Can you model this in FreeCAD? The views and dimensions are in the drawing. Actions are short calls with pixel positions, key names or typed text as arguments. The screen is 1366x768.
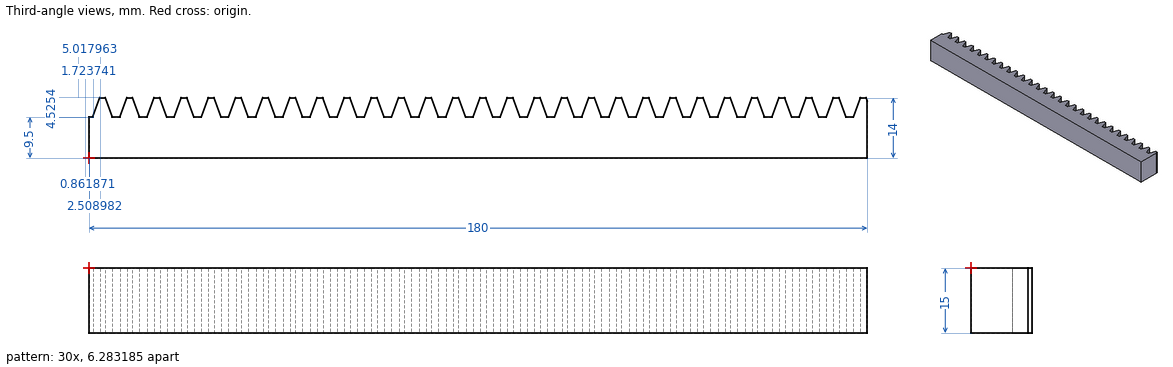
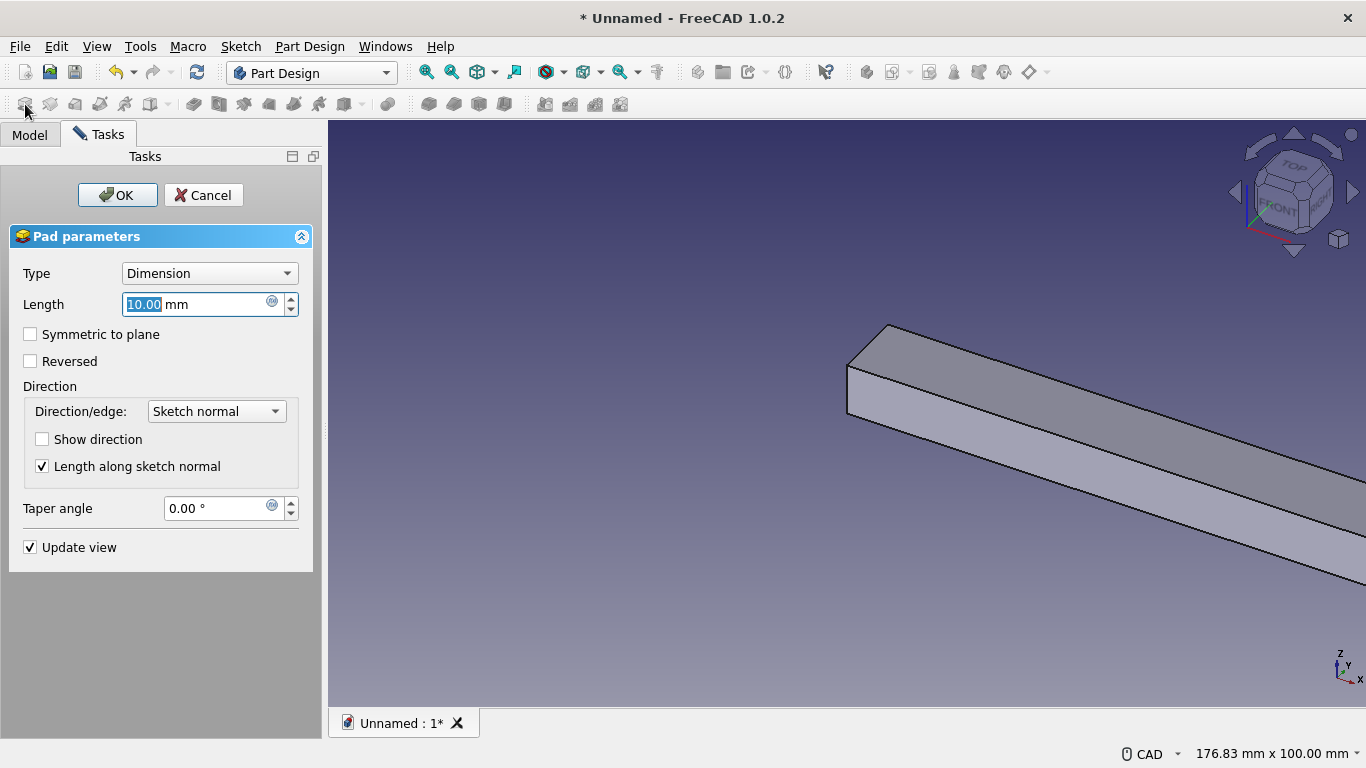
text(15)
key(Tab)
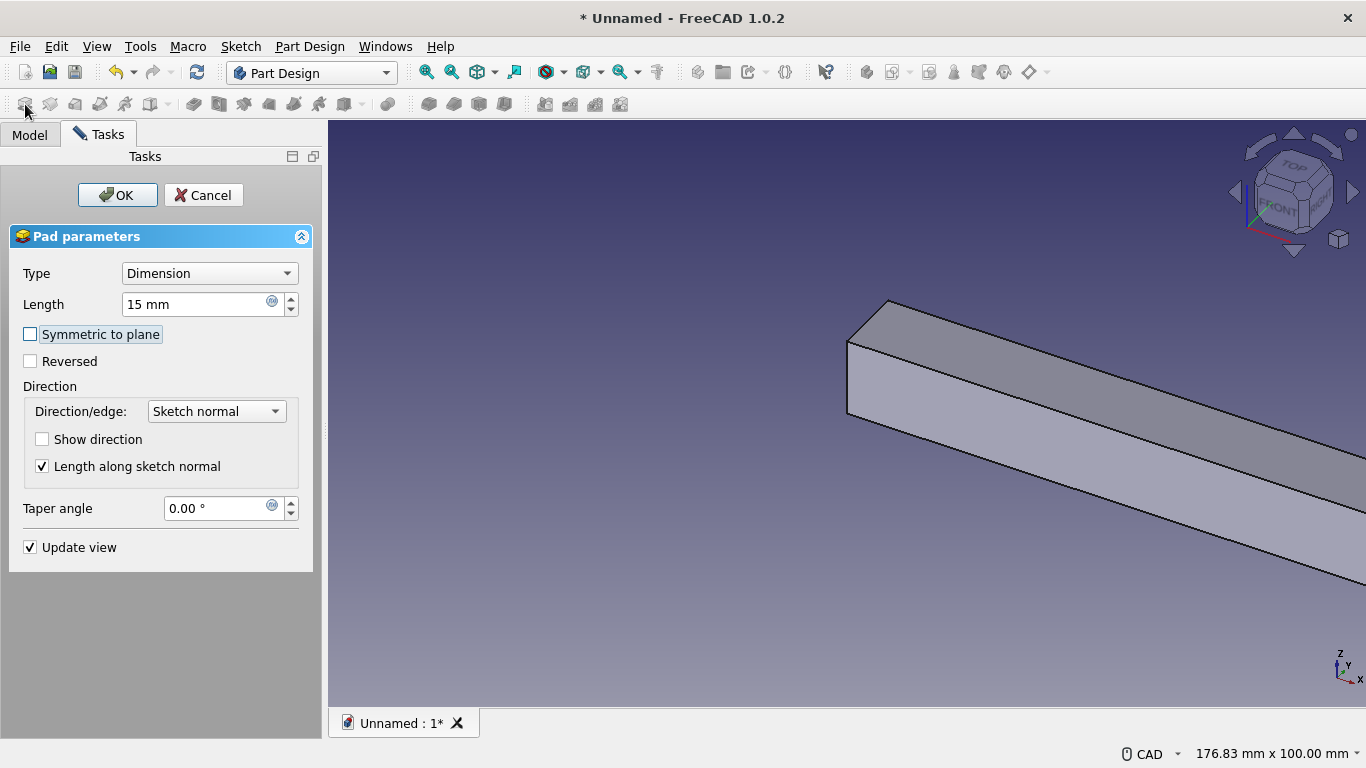
click(31, 361)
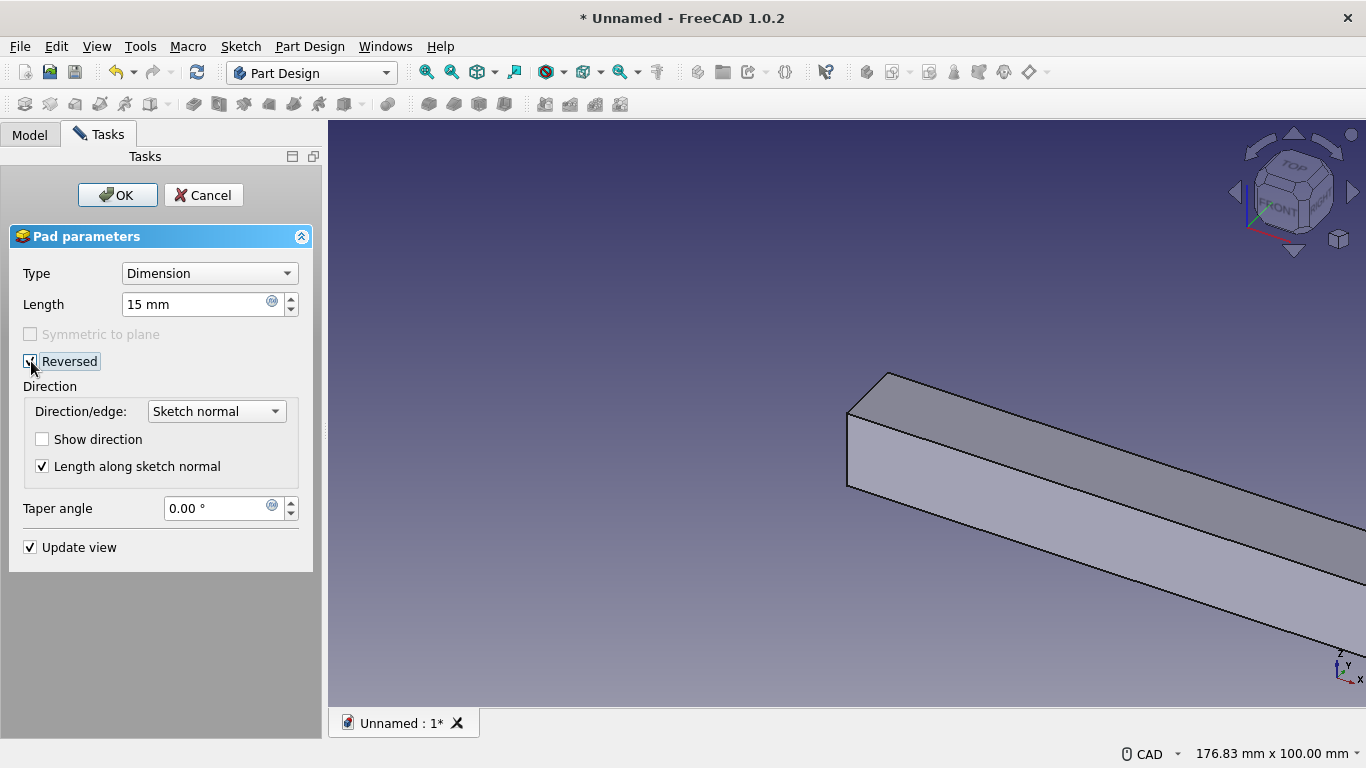
click(118, 195)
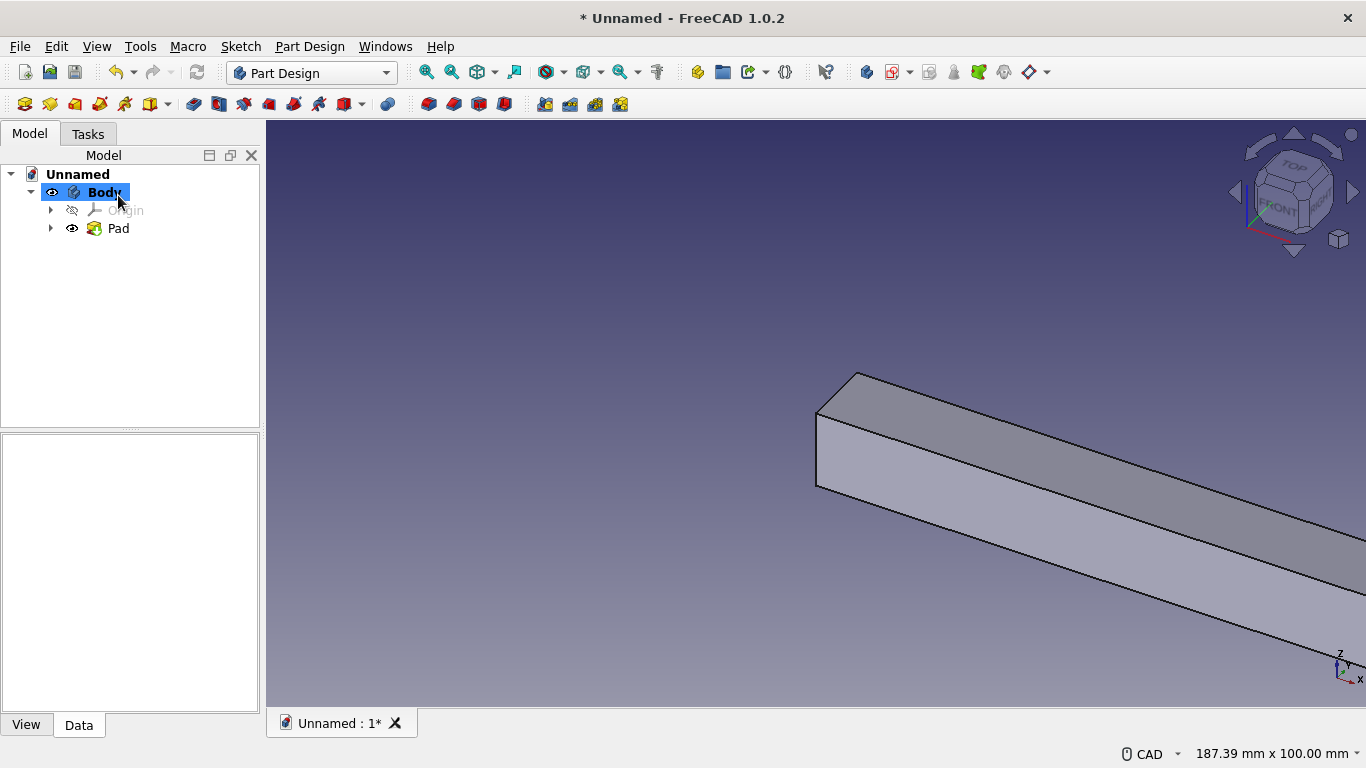
click(427, 72)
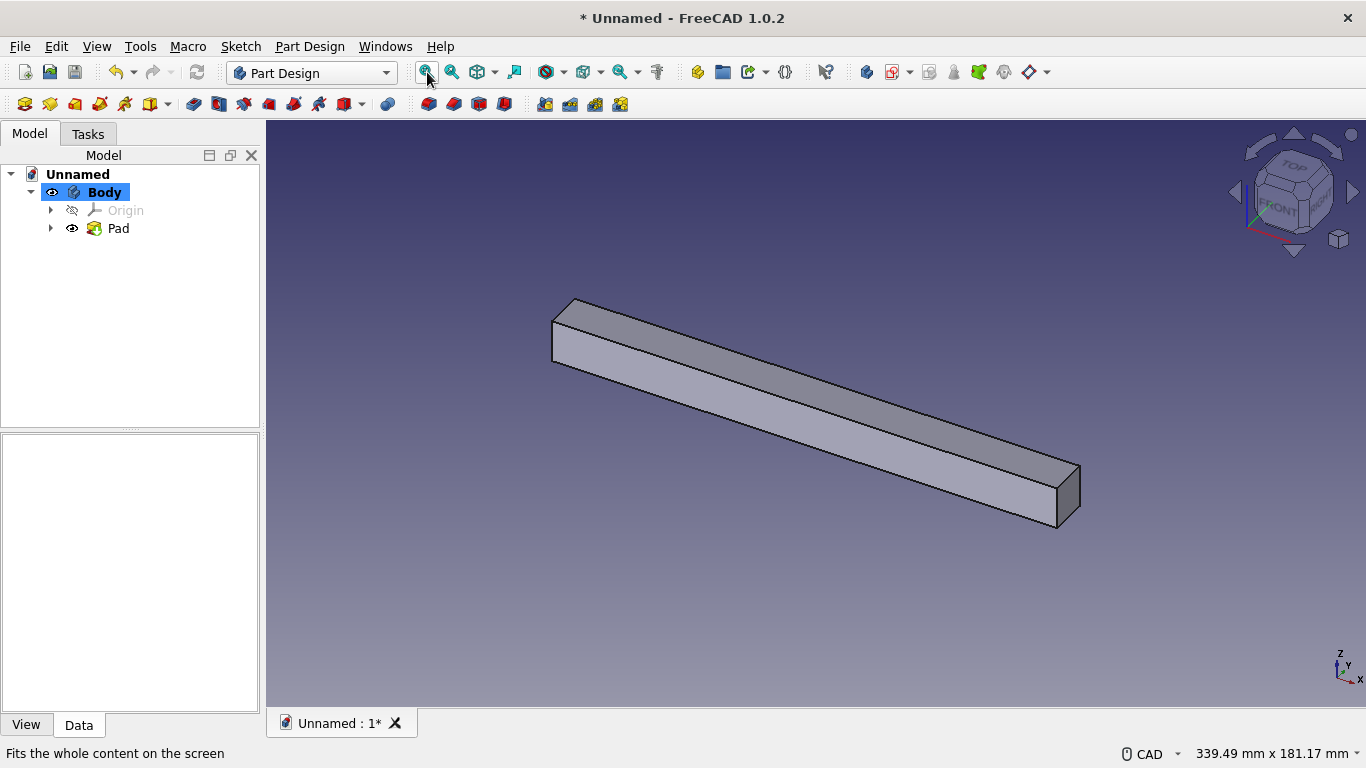
click(1032, 464)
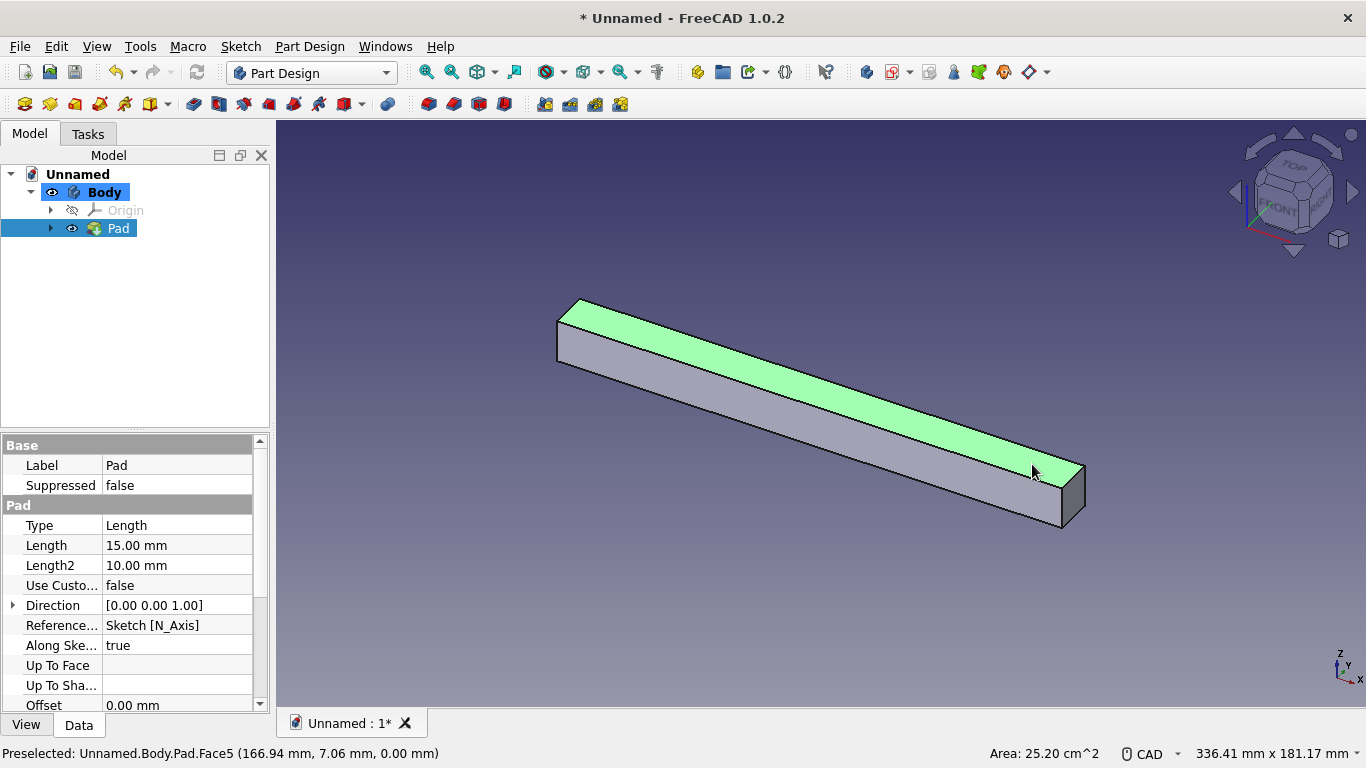
click(892, 72)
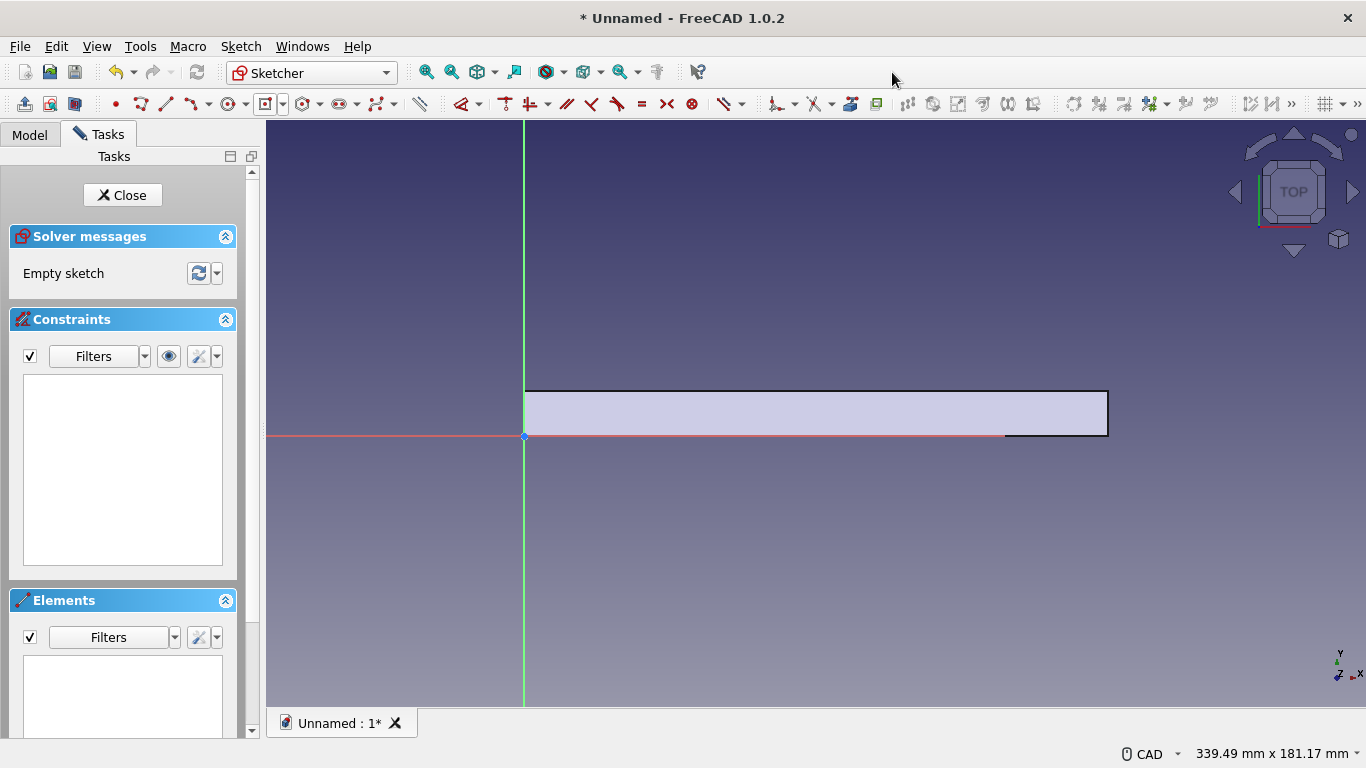
scroll(513, 397, up, 15)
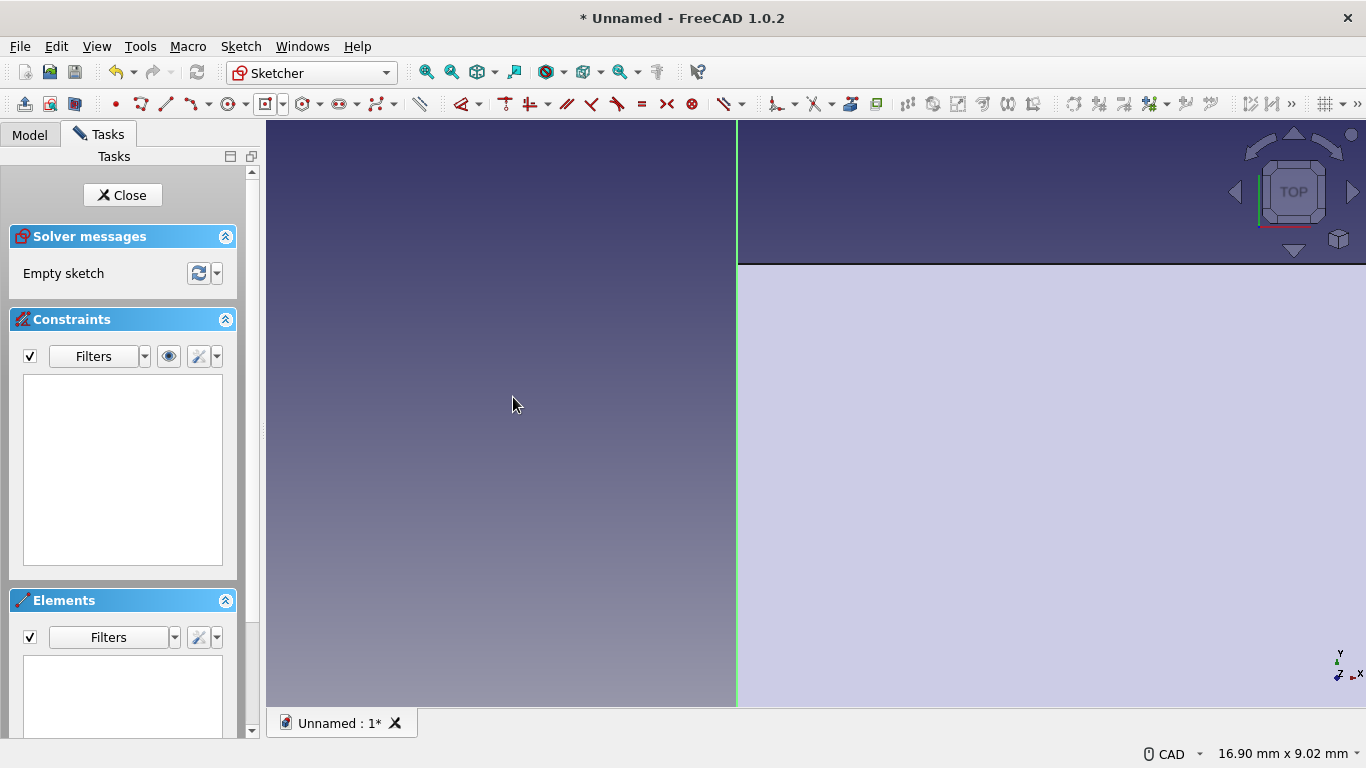
click(141, 104)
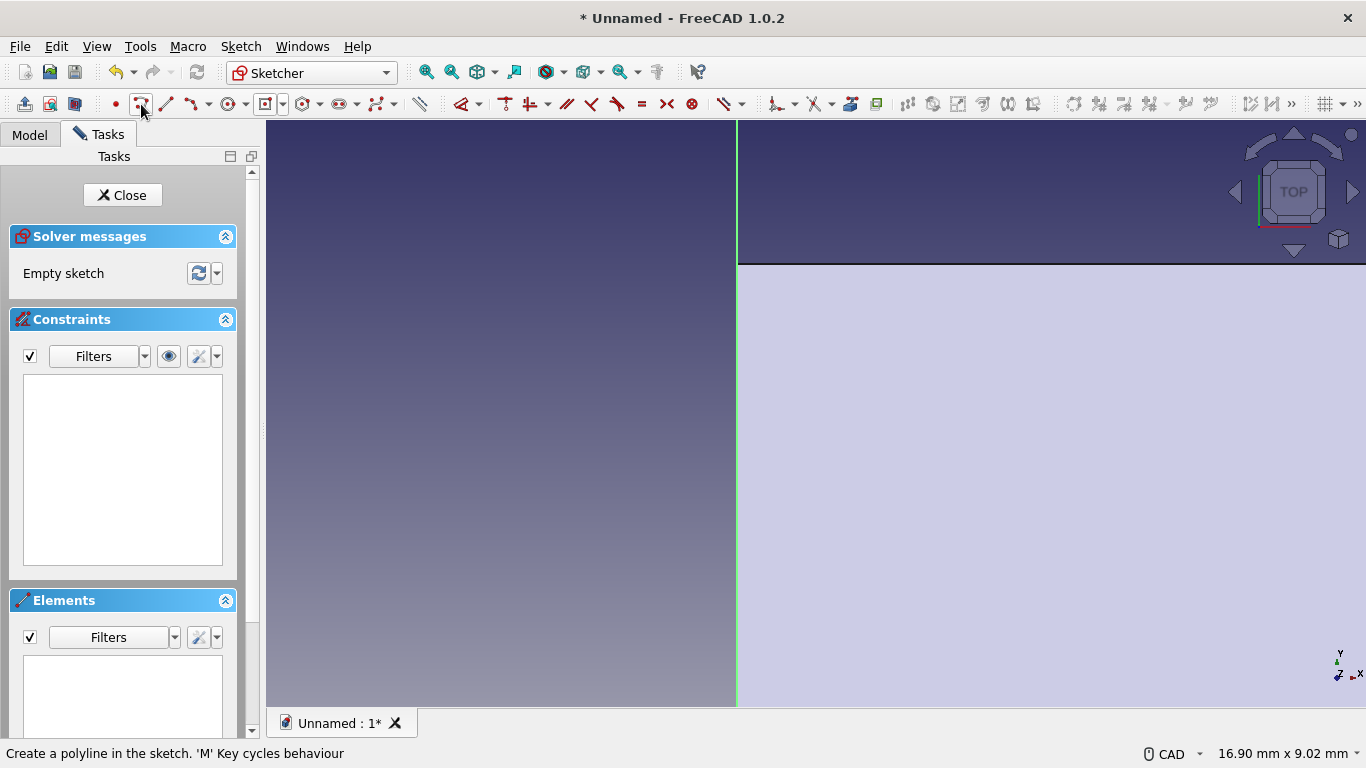
click(681, 557)
click(794, 557)
click(901, 262)
click(574, 262)
click(681, 558)
key(Escape)
key(Escape)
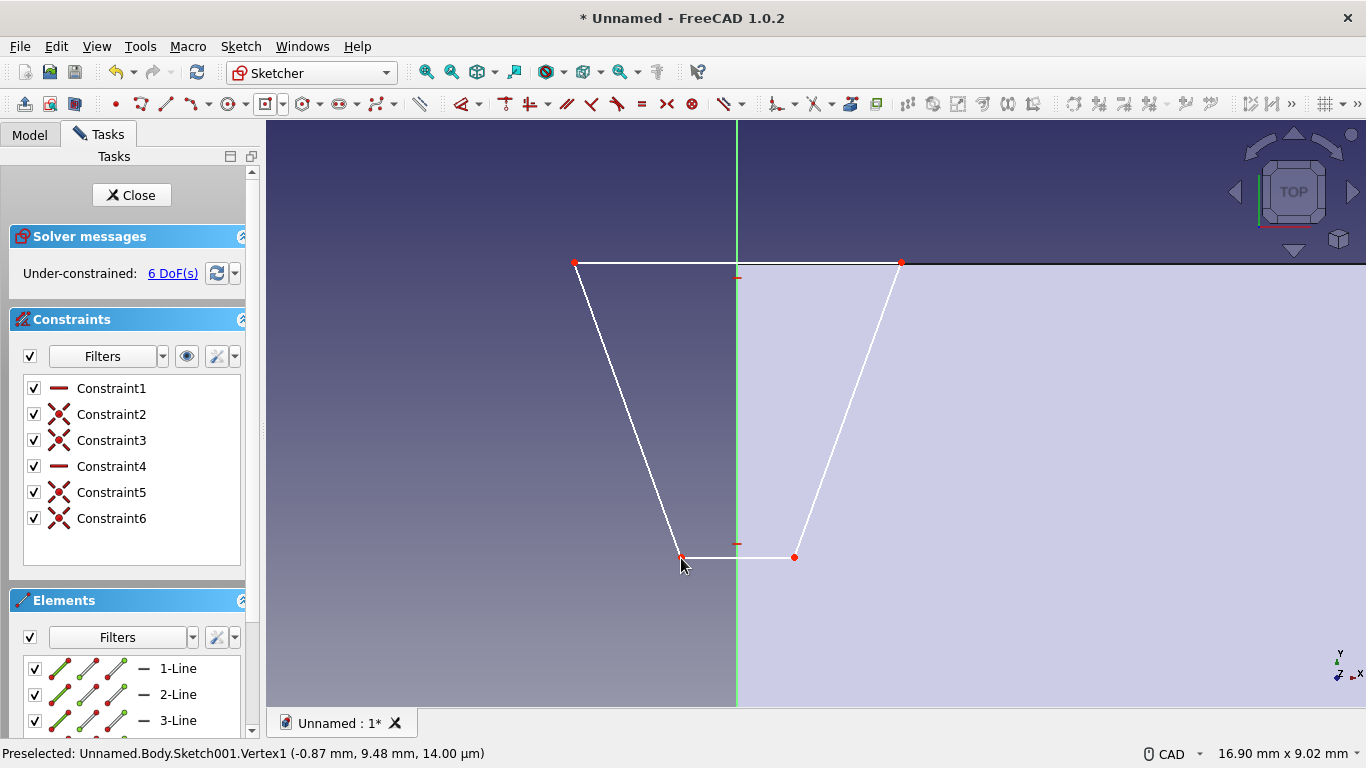
click(460, 104)